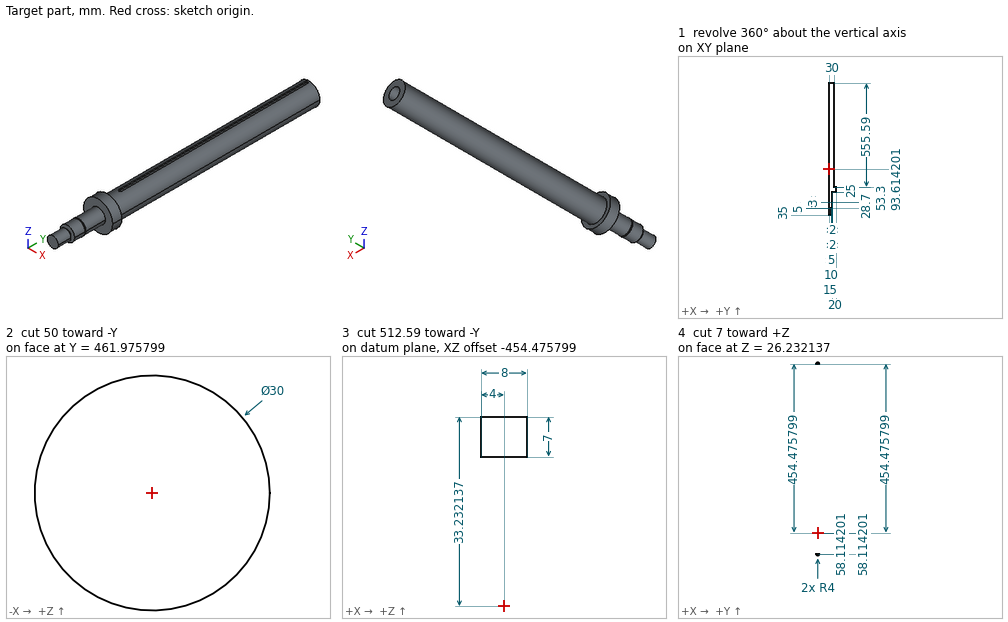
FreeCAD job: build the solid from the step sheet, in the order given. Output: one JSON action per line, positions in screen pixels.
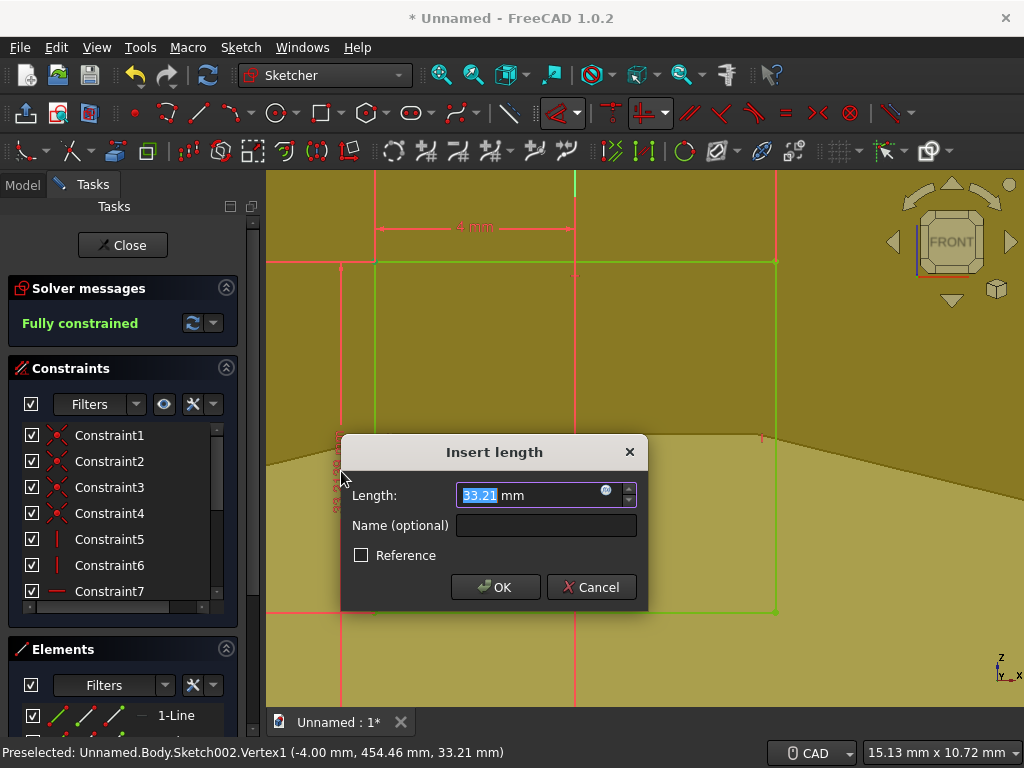
{"action": "type", "text": "33.232137"}
{"action": "key", "text": "Return"}
{"action": "key", "text": "Escape"}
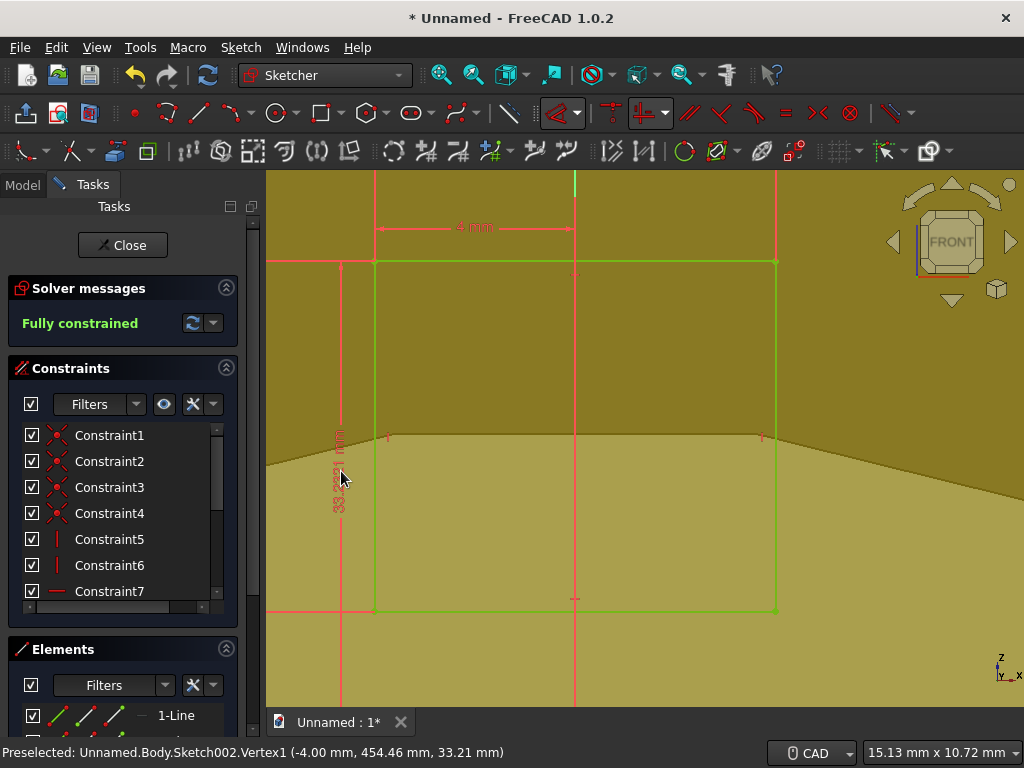
{"action": "left_click", "coordinate": [123, 245]}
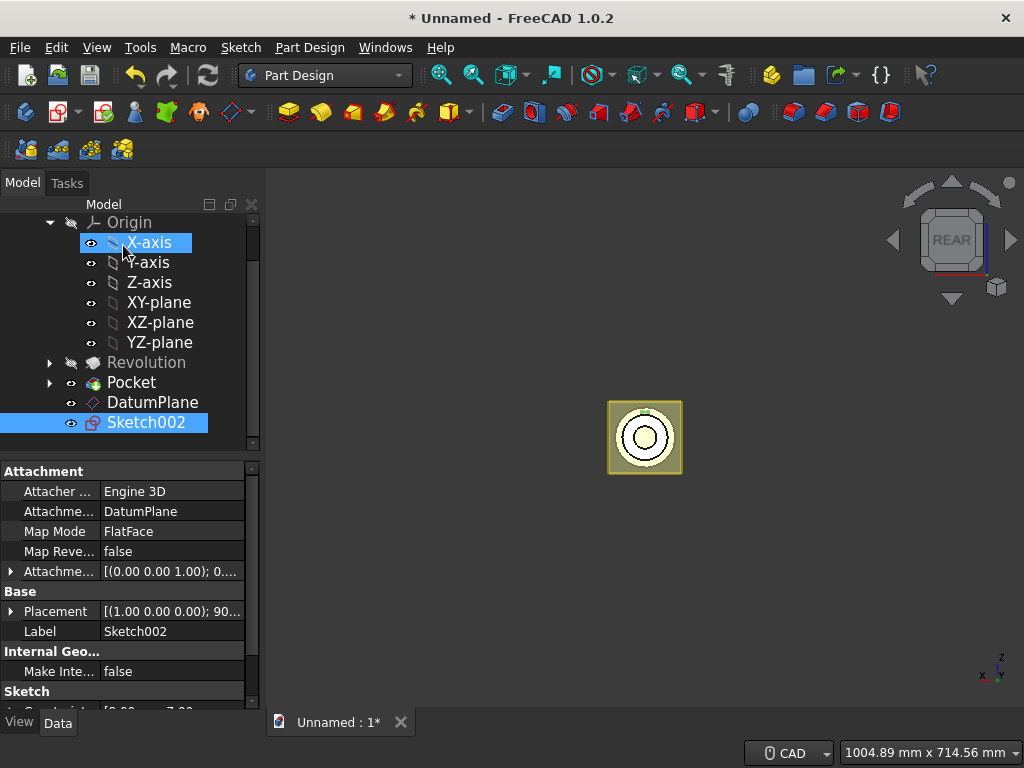
{"action": "left_click", "coordinate": [504, 112]}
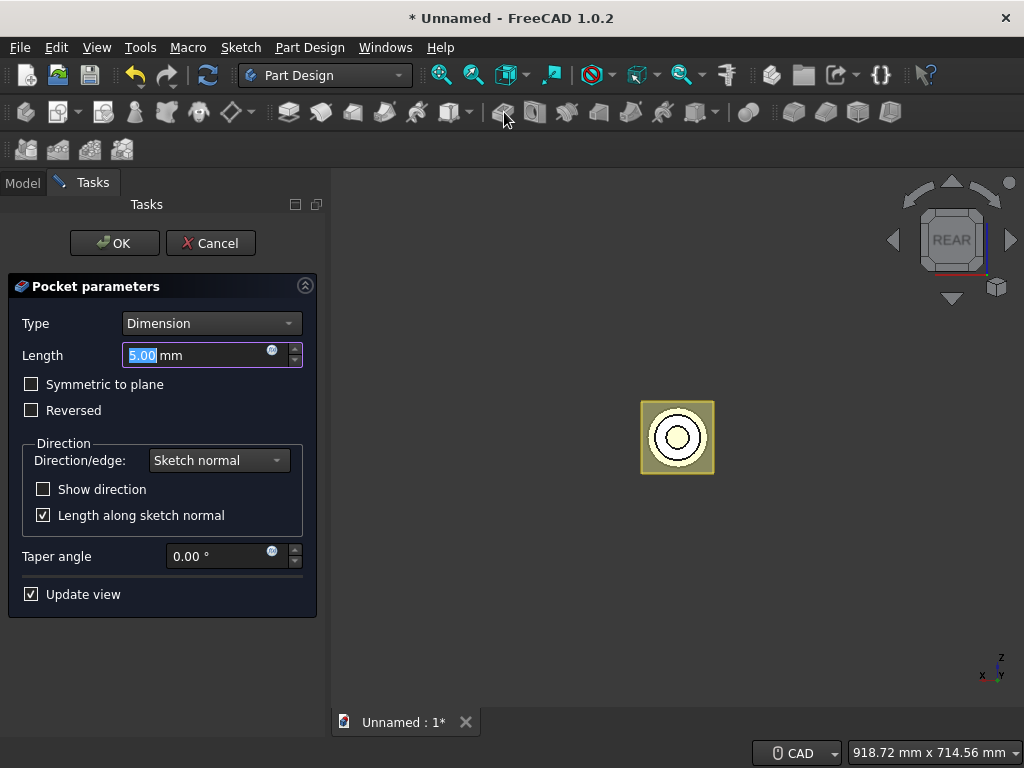
{"action": "type", "text": "512.59"}
{"action": "key", "text": "Tab"}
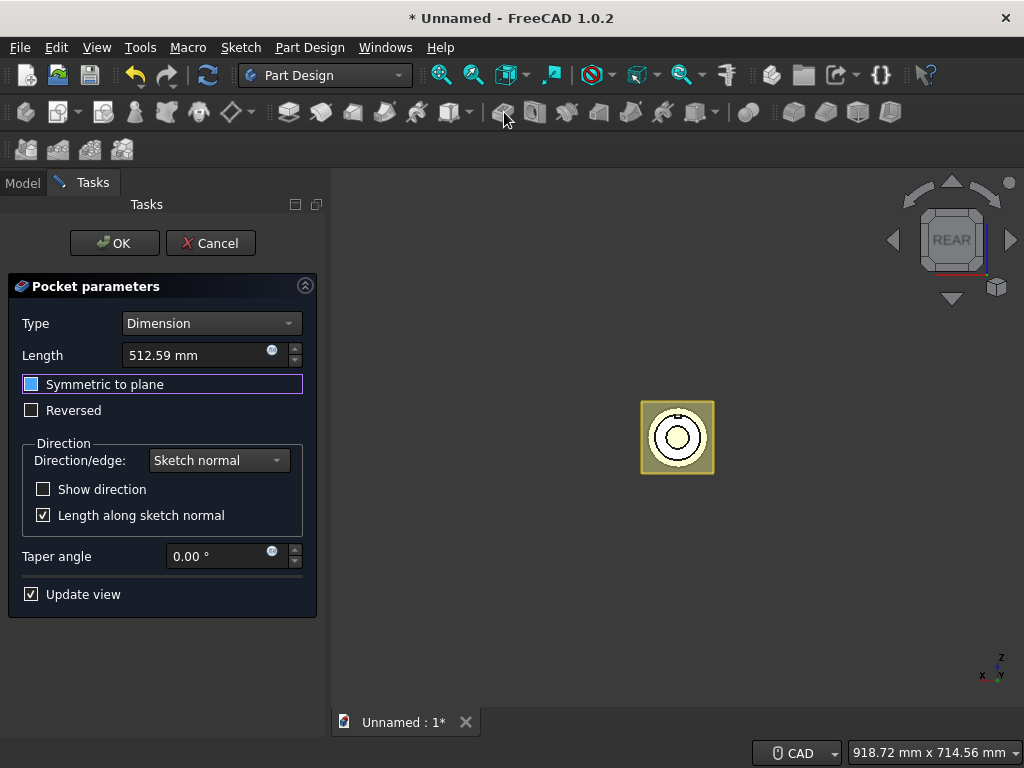
{"action": "left_click", "coordinate": [30, 410]}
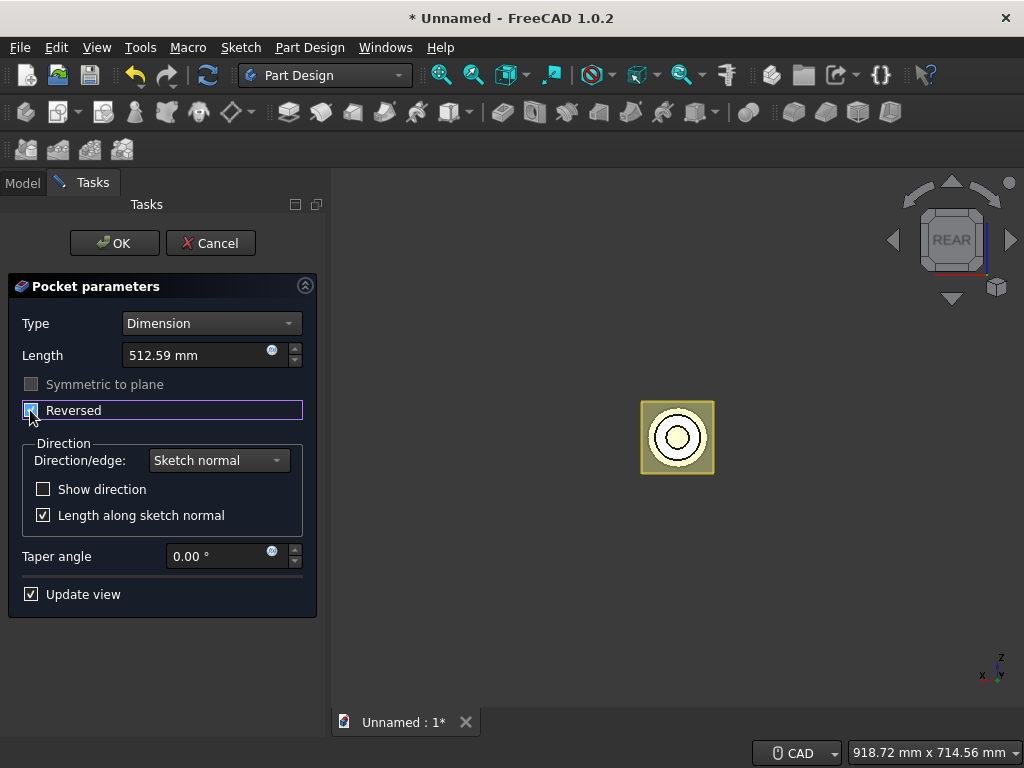
{"action": "left_click", "coordinate": [115, 243]}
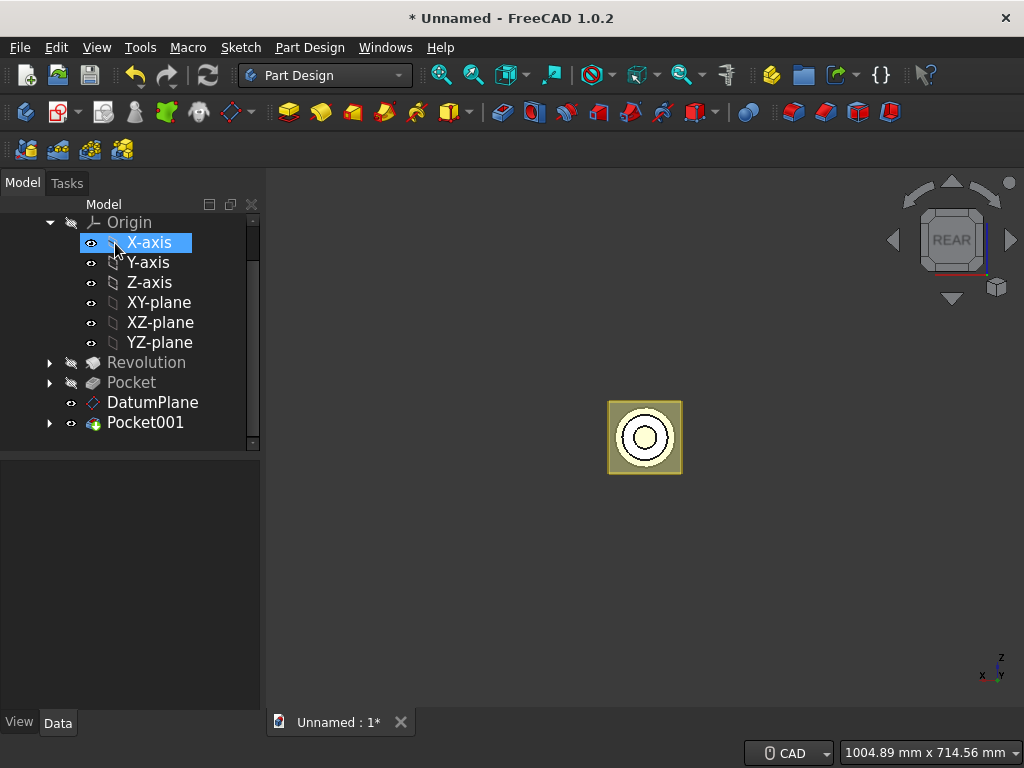
{"action": "left_click", "coordinate": [116, 403]}
{"action": "key", "text": "space"}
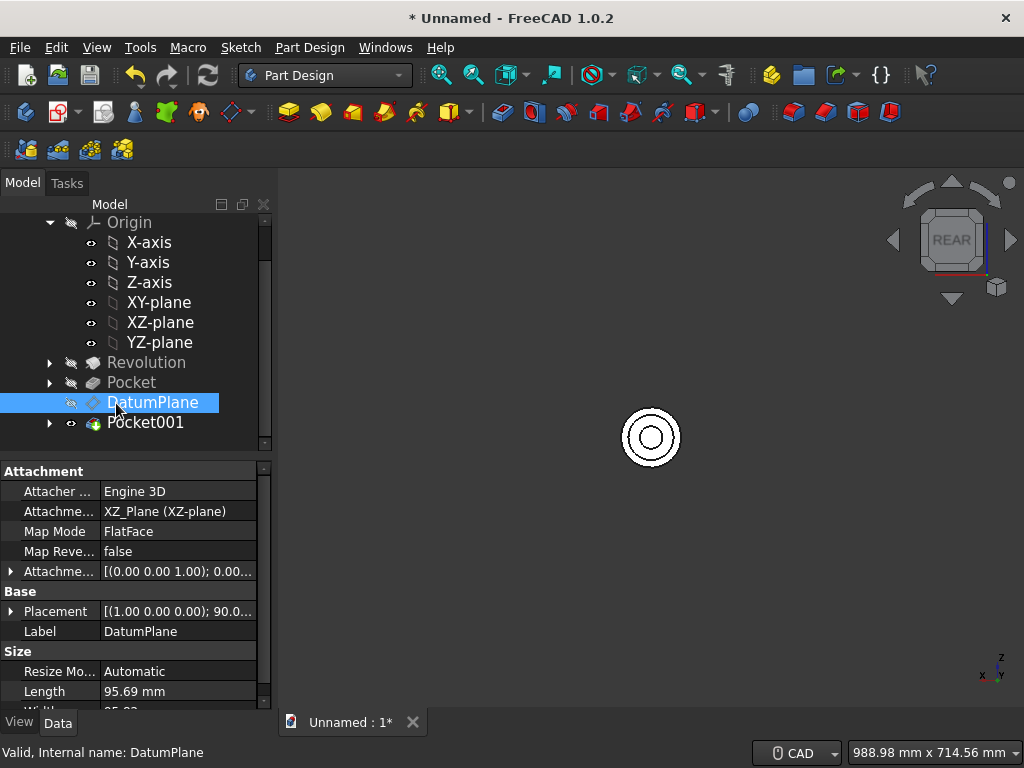
{"action": "key", "text": "v f"}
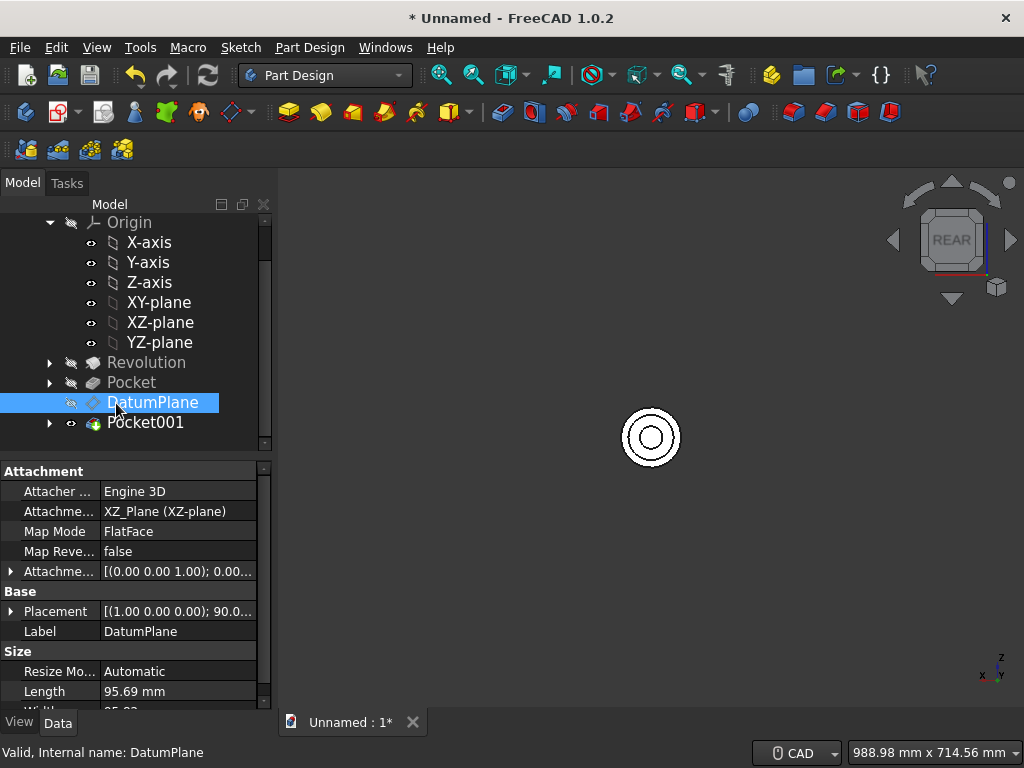
{"action": "key", "text": "0"}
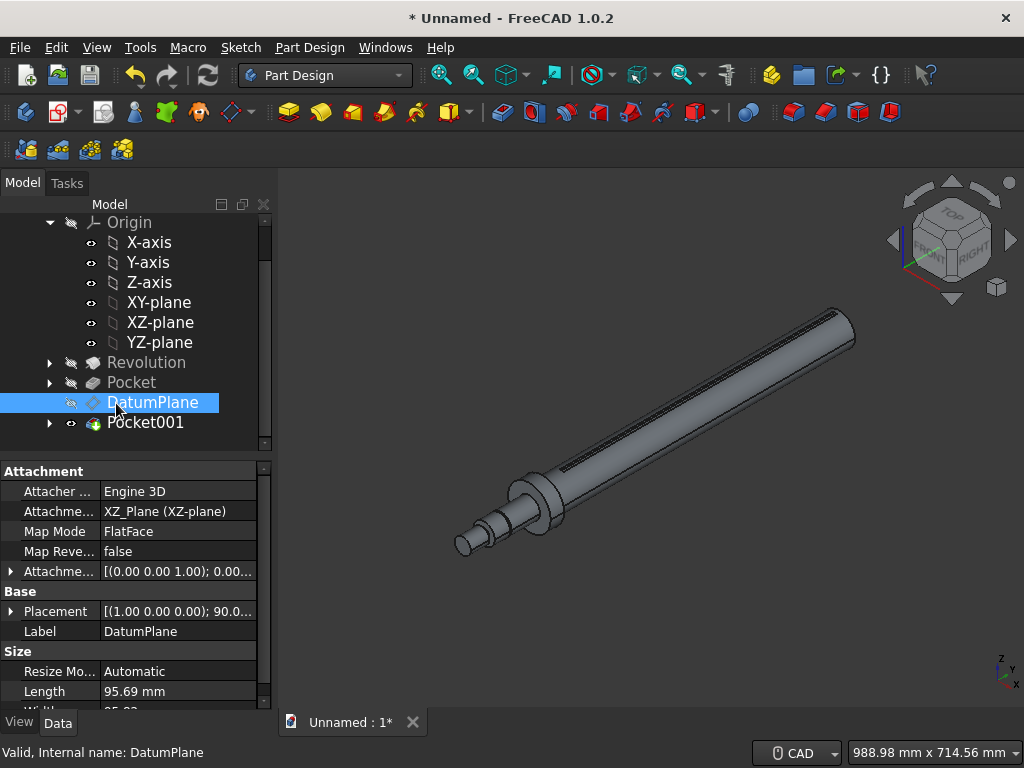
{"action": "scroll", "coordinate": [816, 325], "scroll_direction": "up", "scroll_amount": 7}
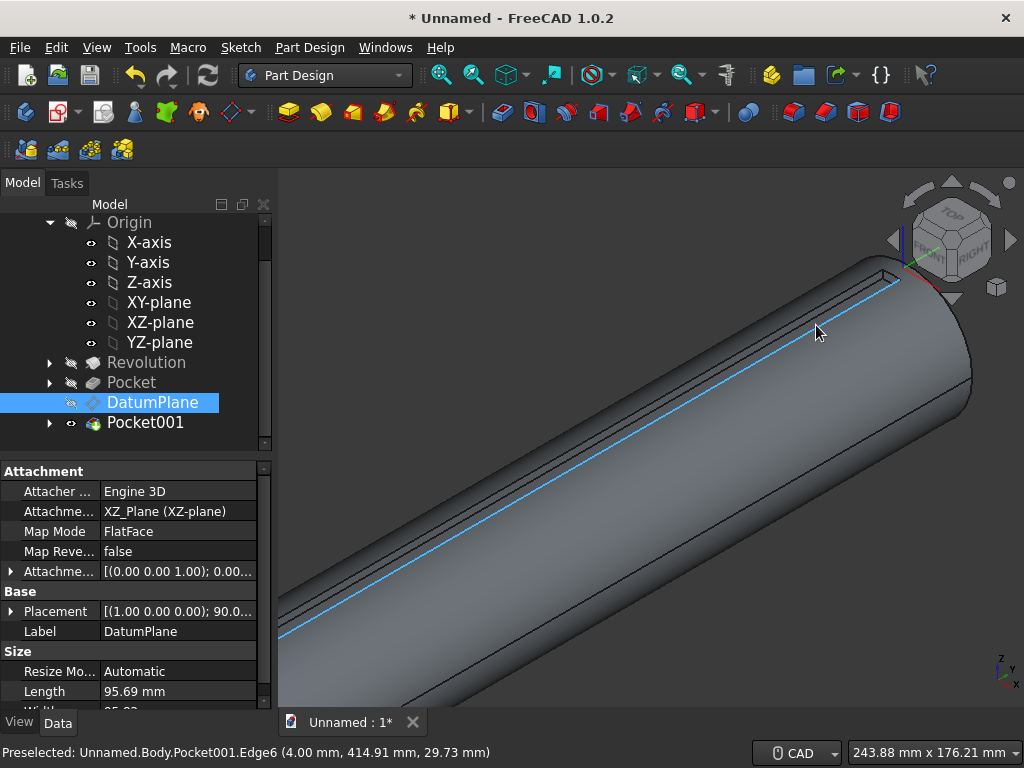
{"action": "left_click", "coordinate": [442, 76]}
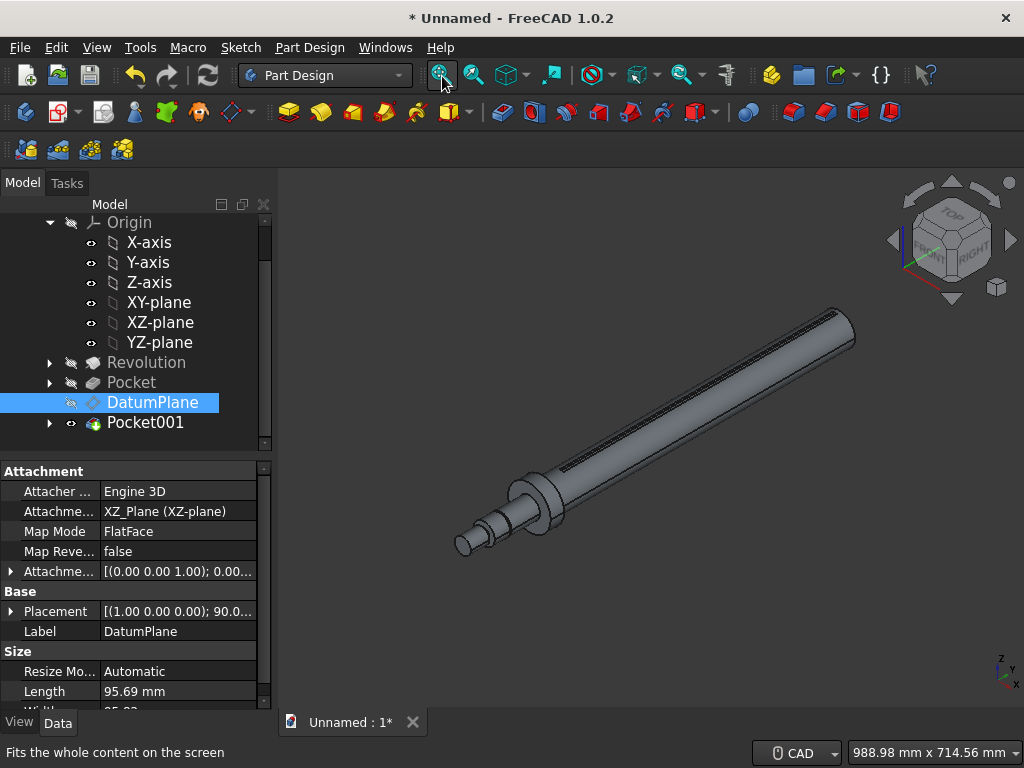
{"action": "key", "text": "2"}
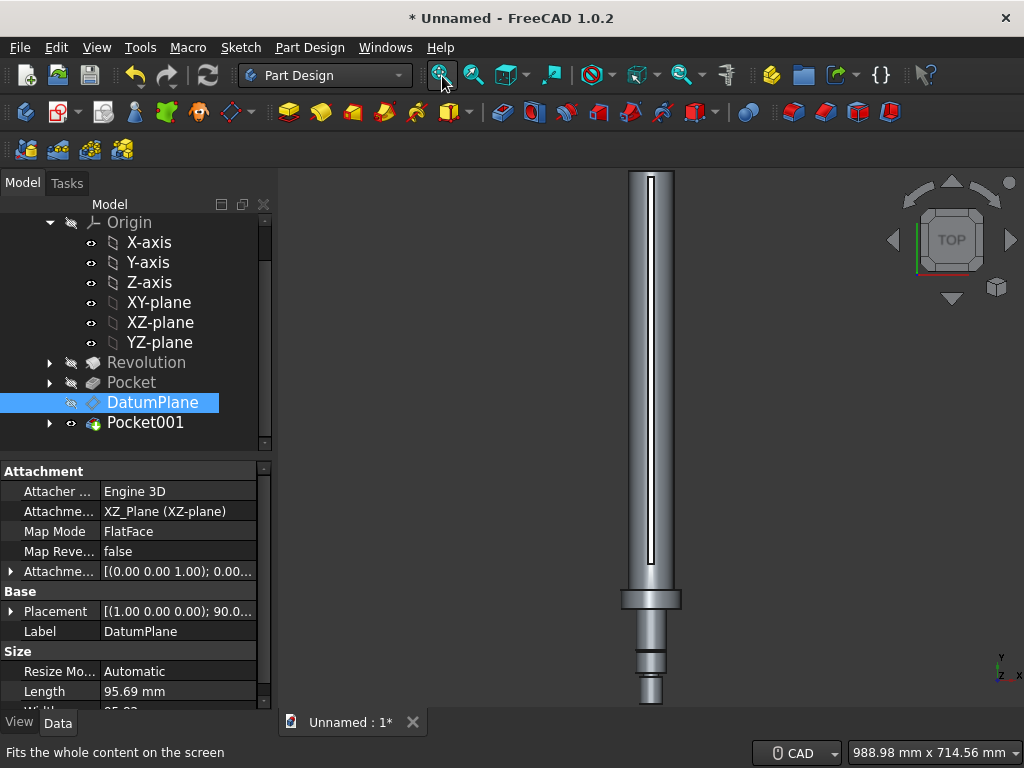
{"action": "scroll", "coordinate": [651, 204], "scroll_direction": "up", "scroll_amount": 7}